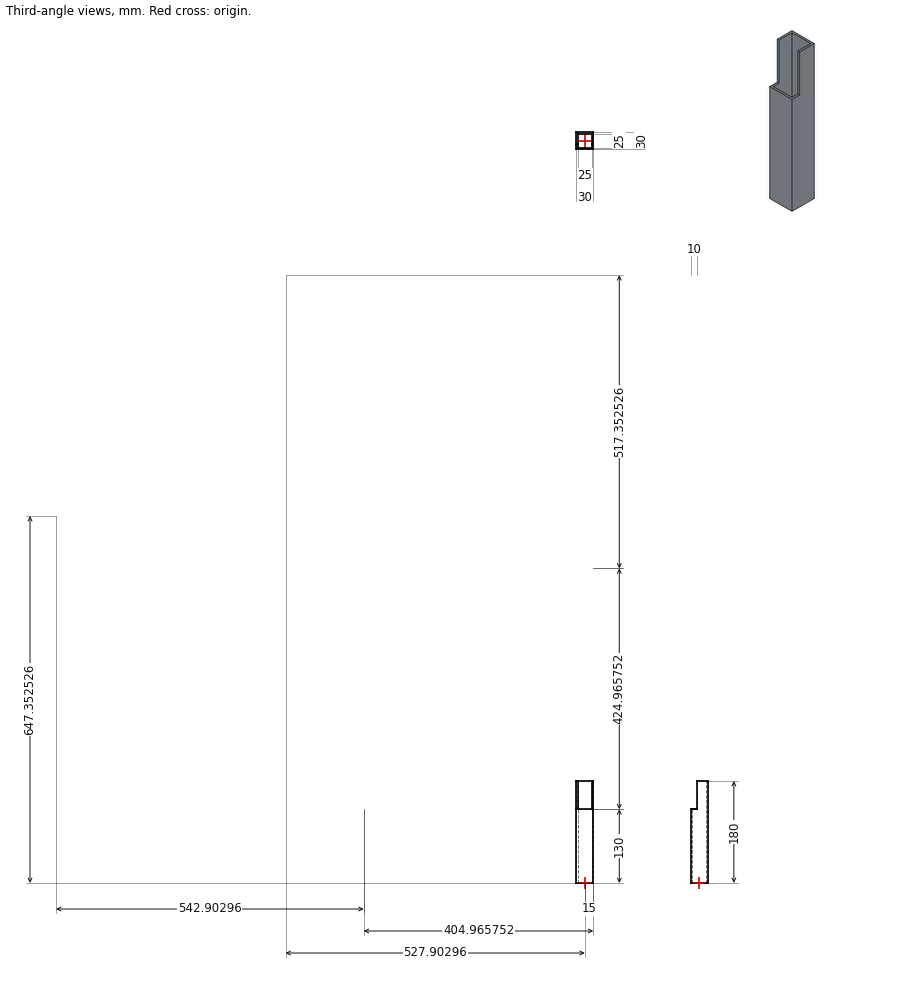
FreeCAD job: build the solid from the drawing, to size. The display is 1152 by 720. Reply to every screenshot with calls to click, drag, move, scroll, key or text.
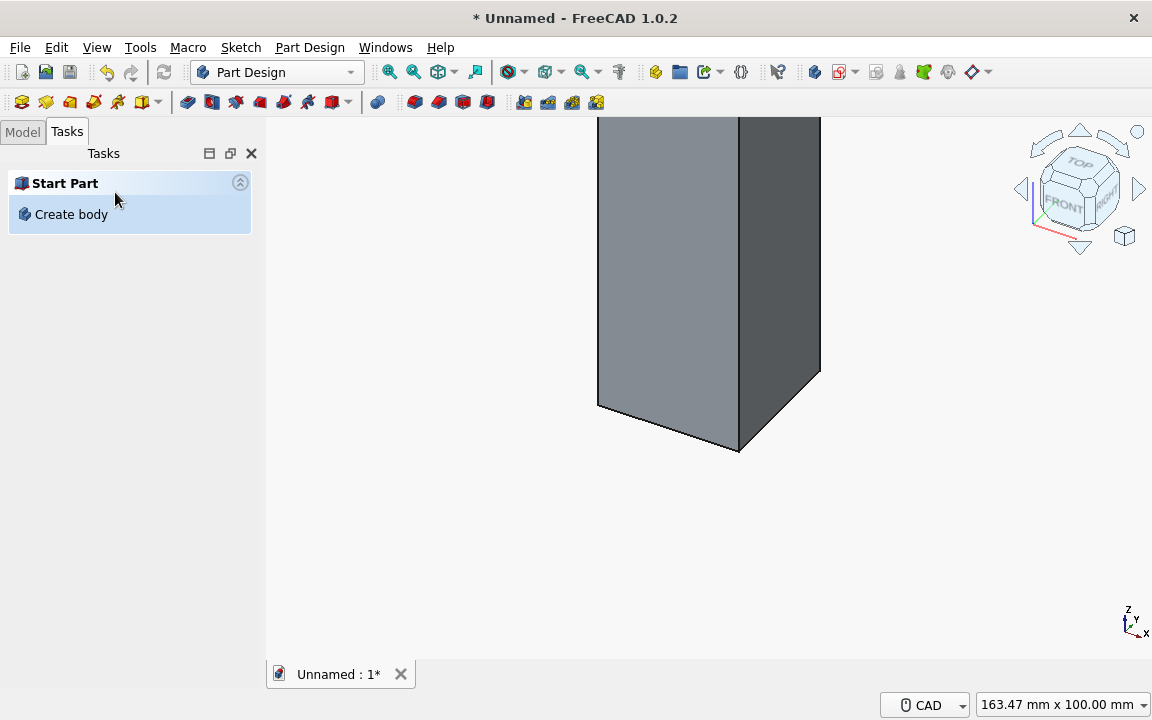
key(v)
key(f)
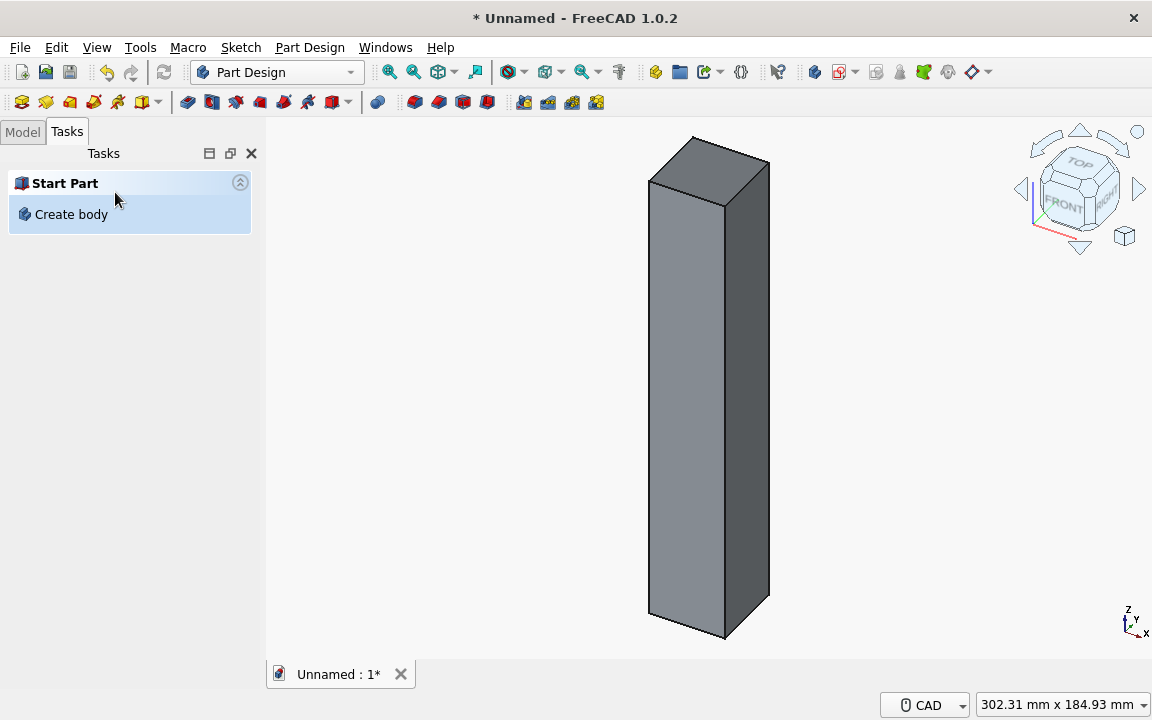
click(840, 72)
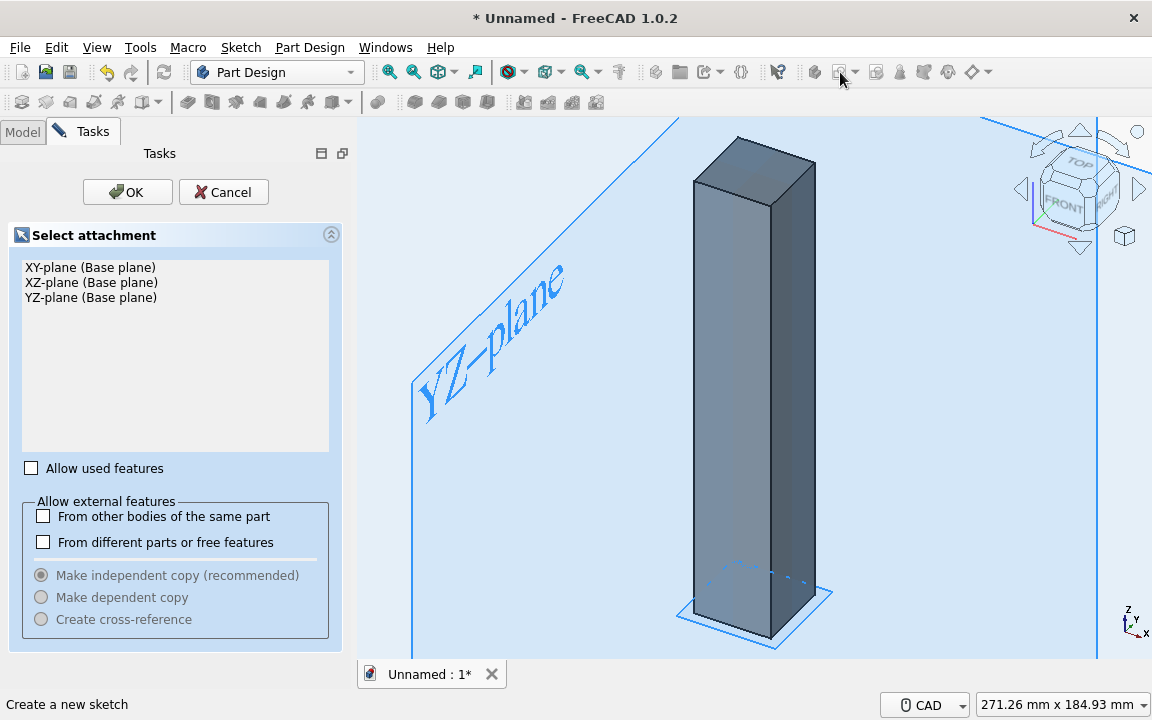
click(82, 268)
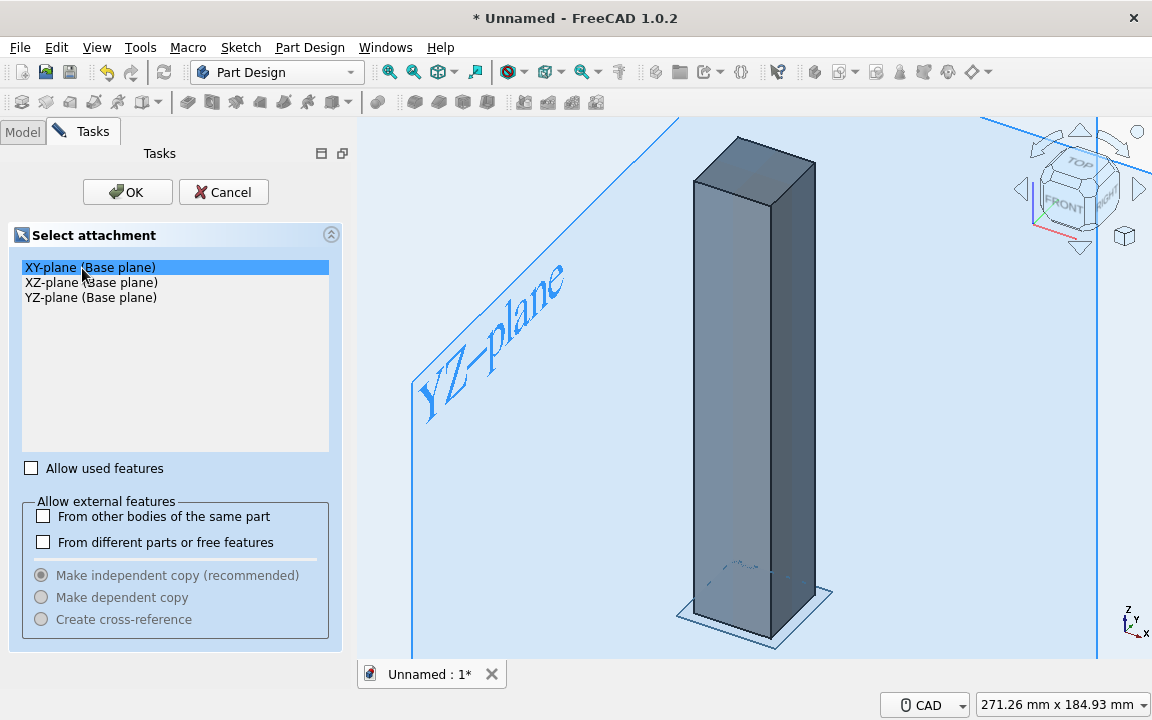
click(128, 192)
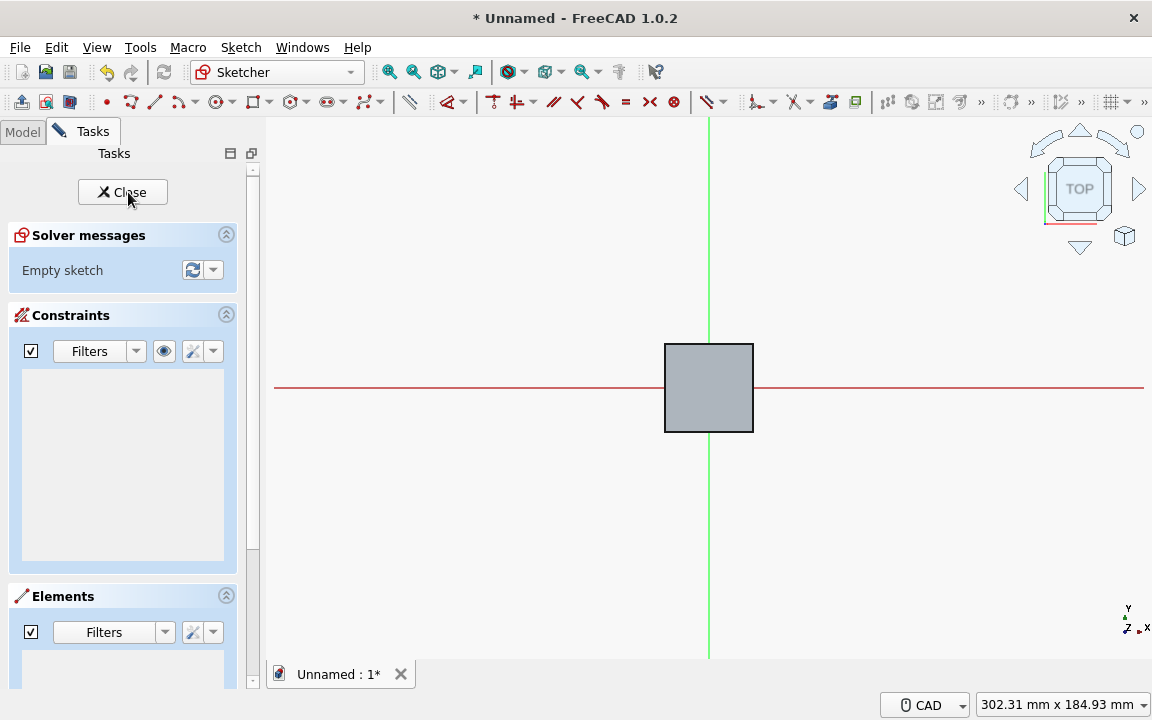
key(q)
key(s)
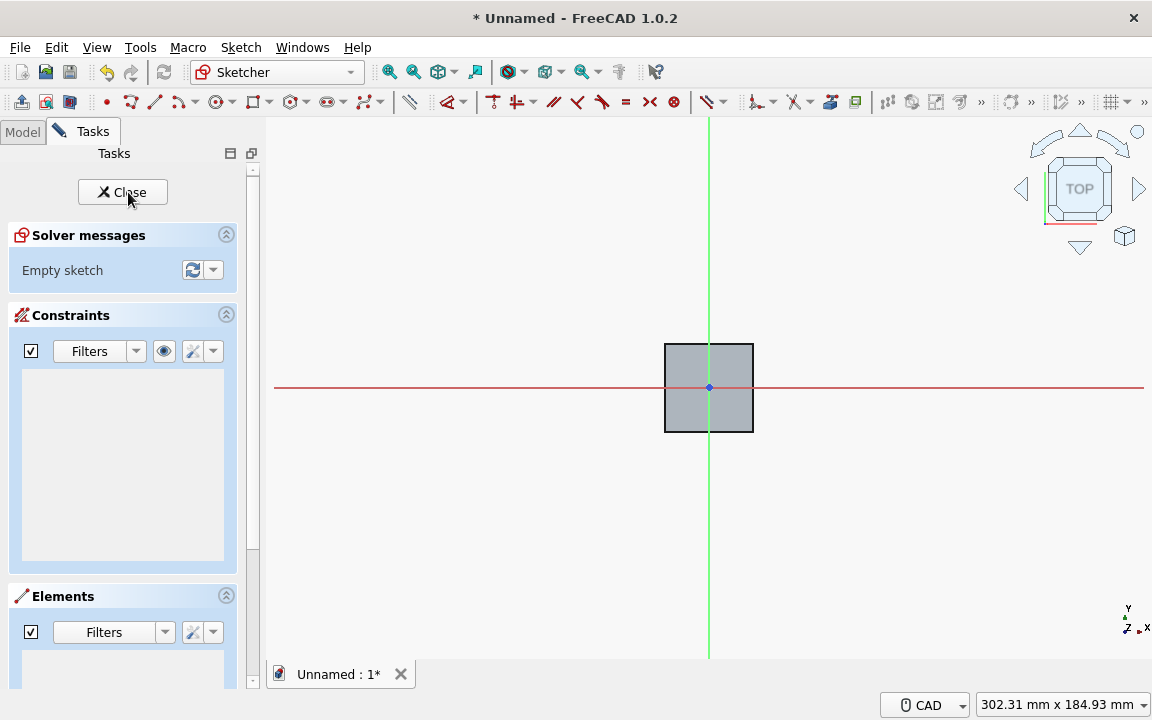
scroll(726, 388, up, 8)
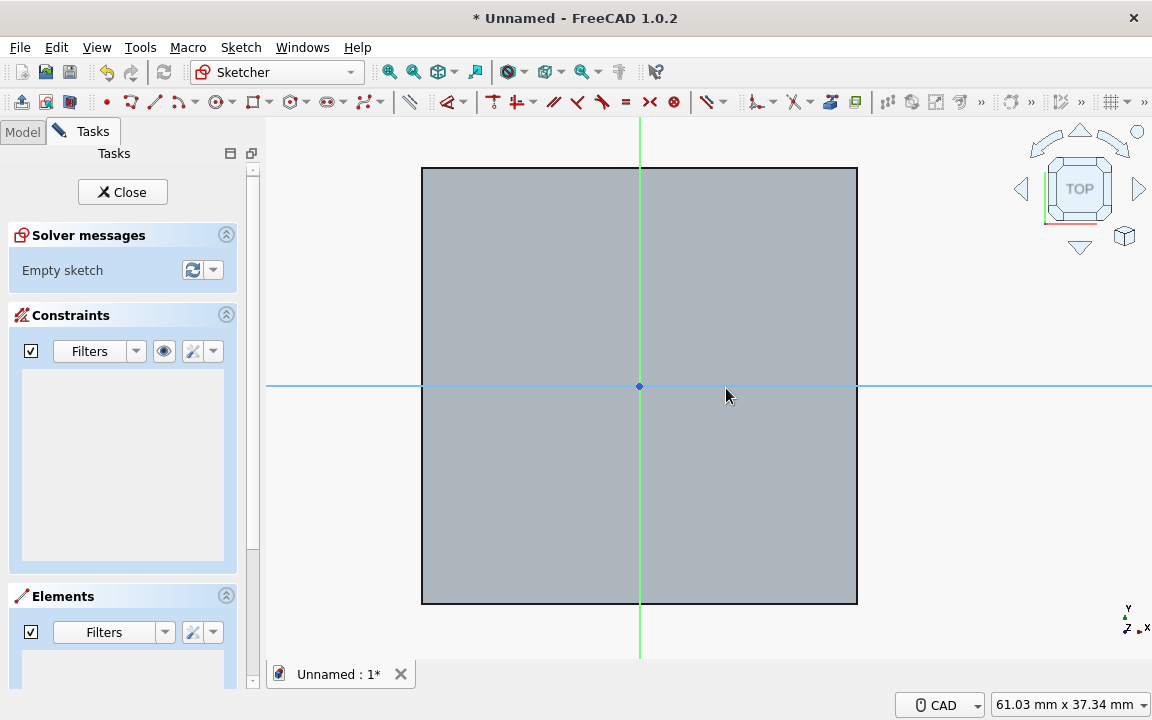
key(g)
key(v)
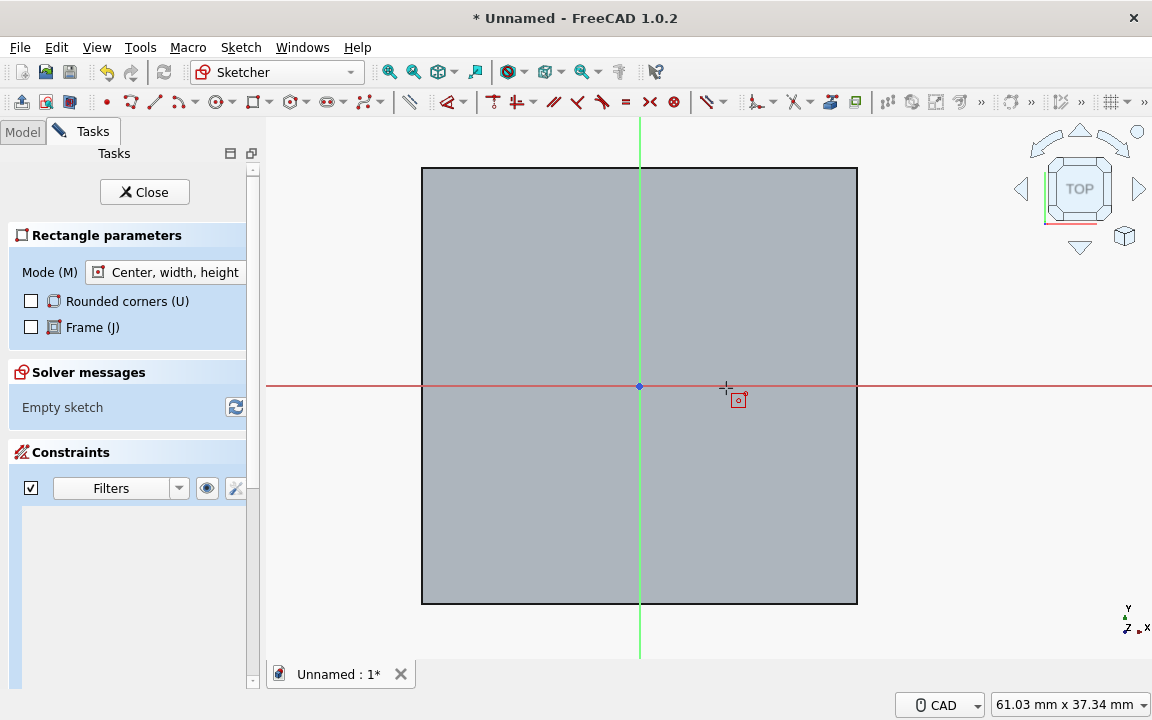
click(640, 386)
move(821, 205)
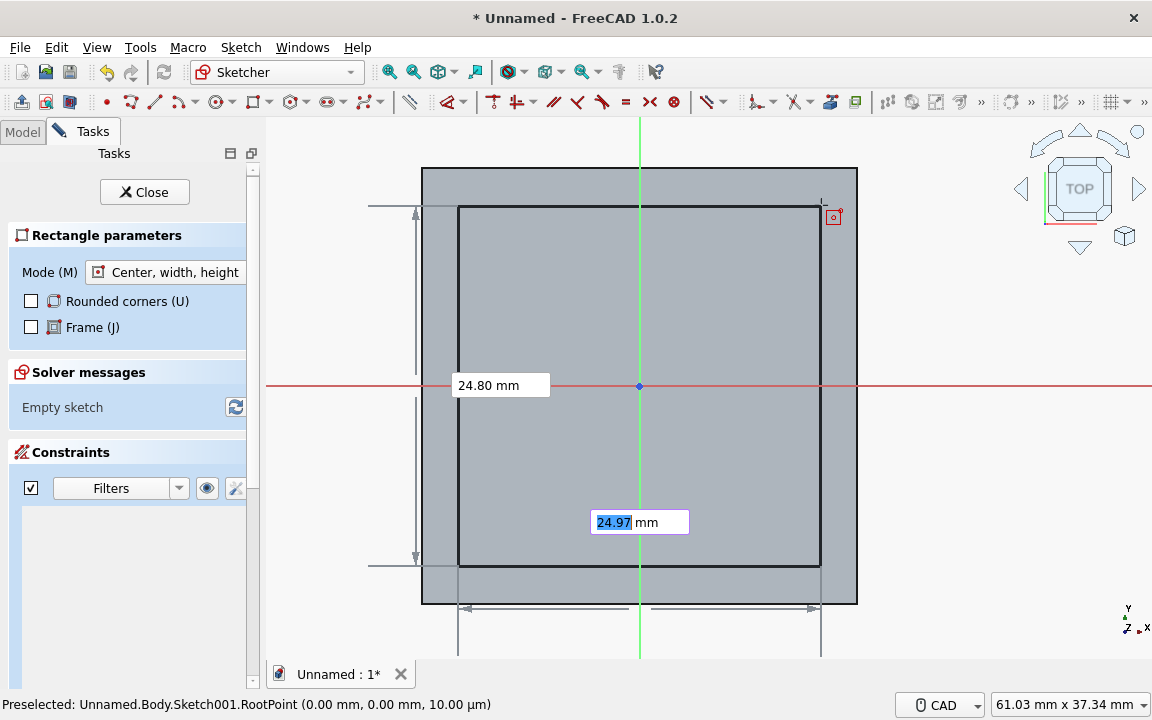
text(25)
key(Tab)
text(25)
key(Return)
key(Escape)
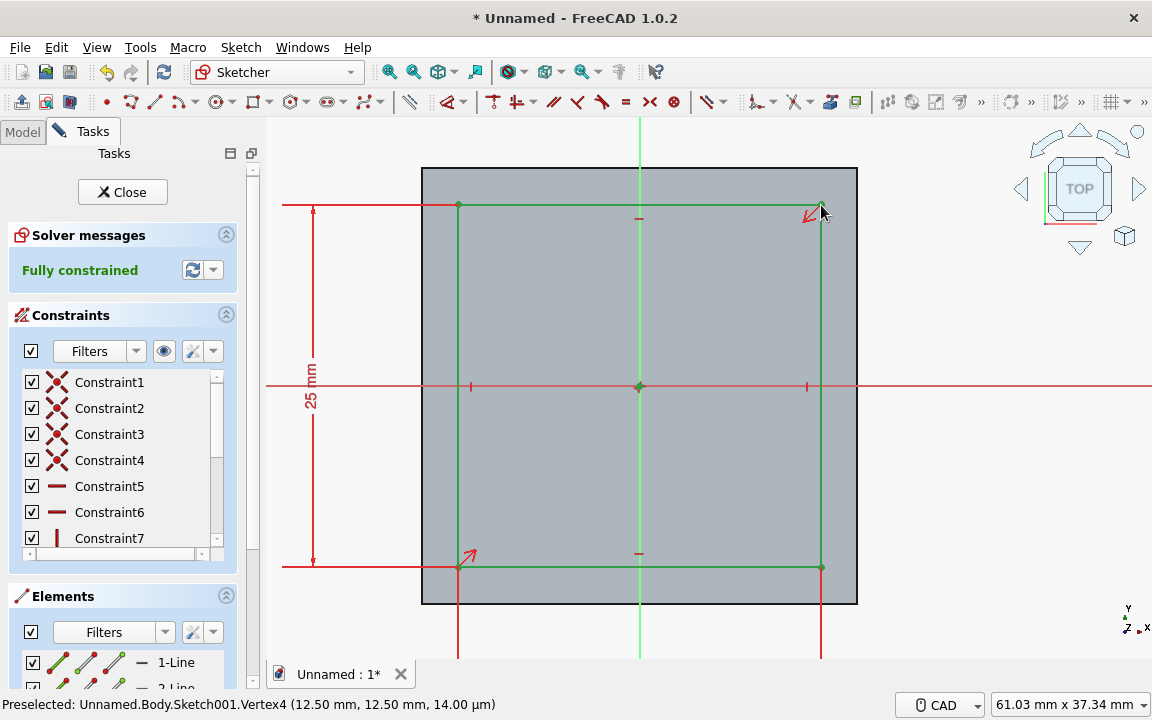
click(123, 192)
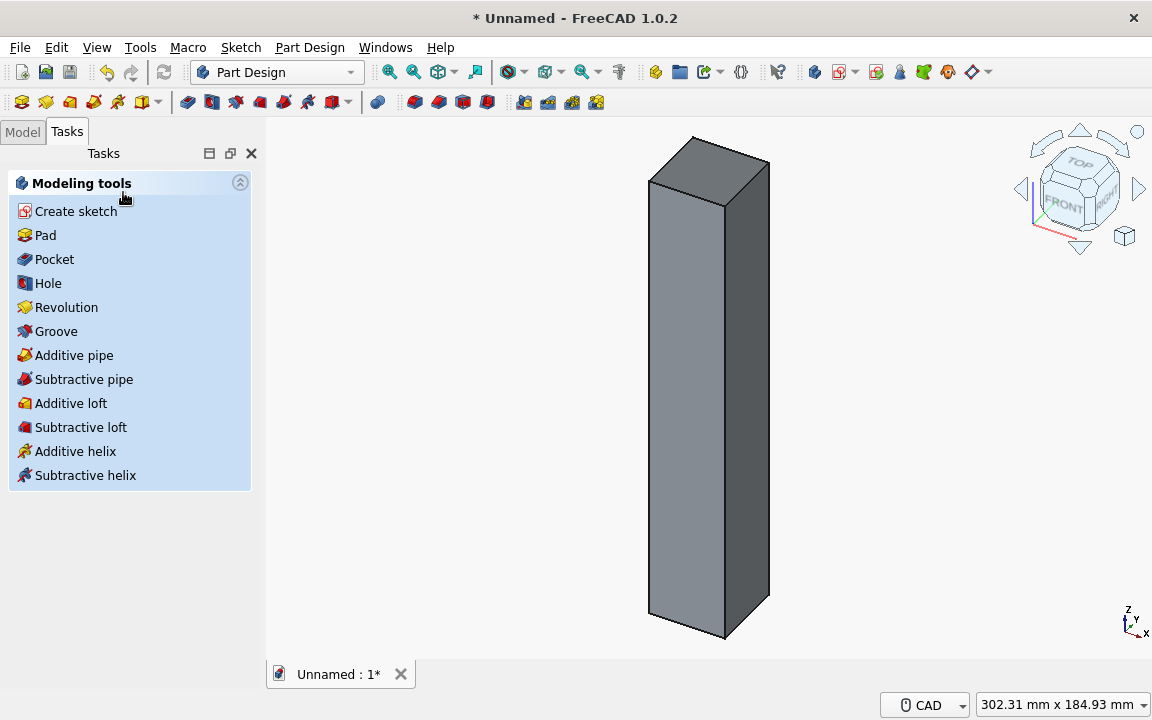
click(188, 102)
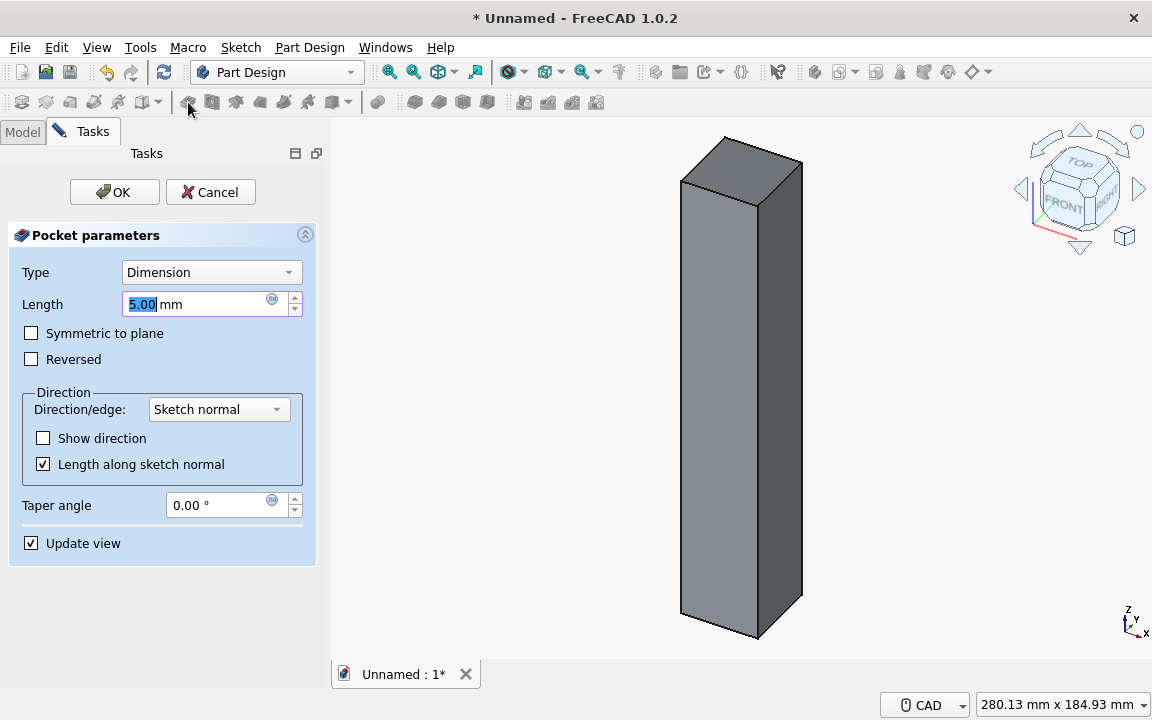
click(212, 272)